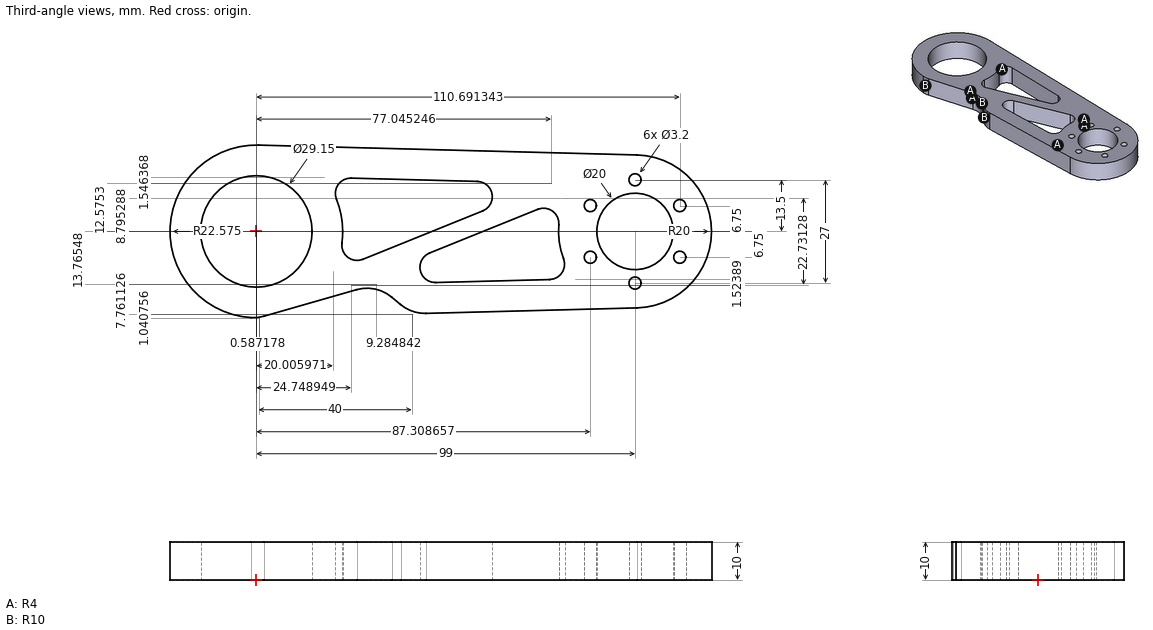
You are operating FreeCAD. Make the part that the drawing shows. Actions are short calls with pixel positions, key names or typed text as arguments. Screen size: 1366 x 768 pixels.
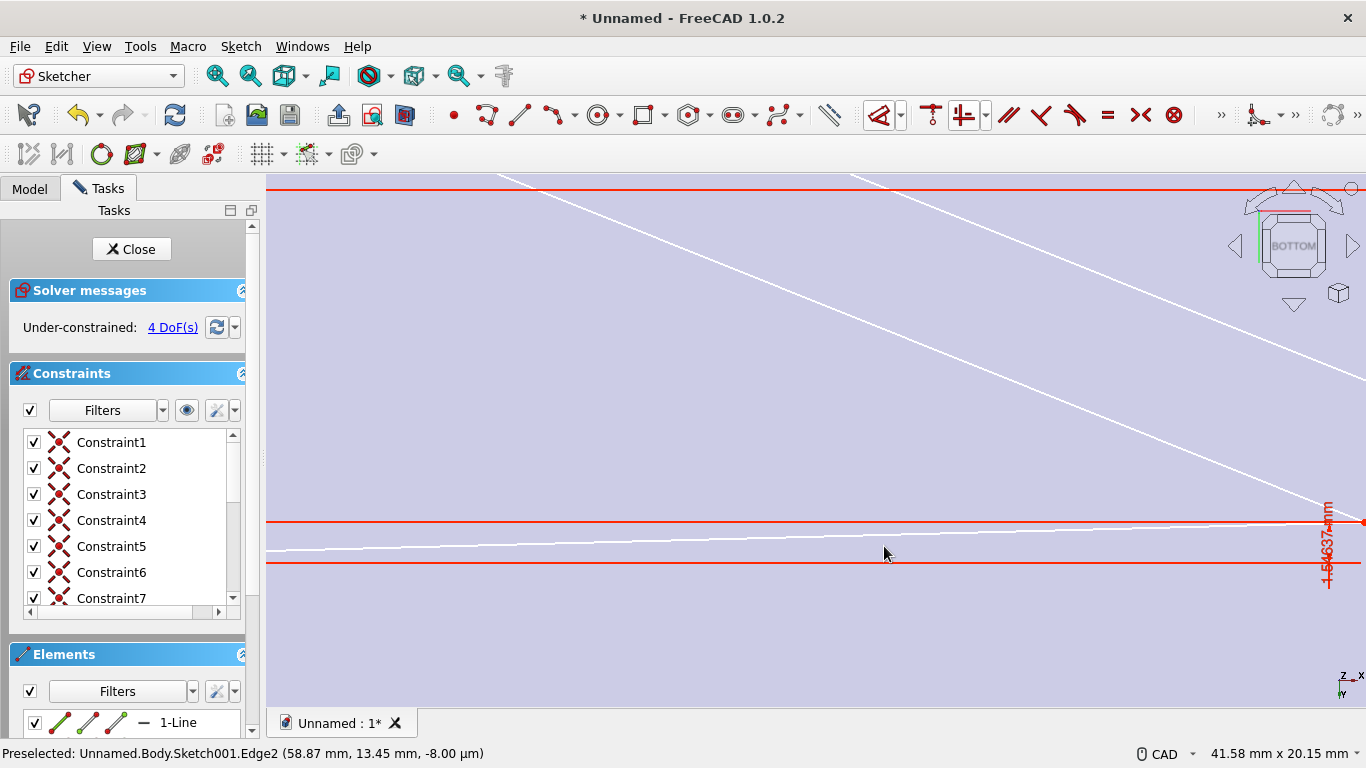
click(1023, 243)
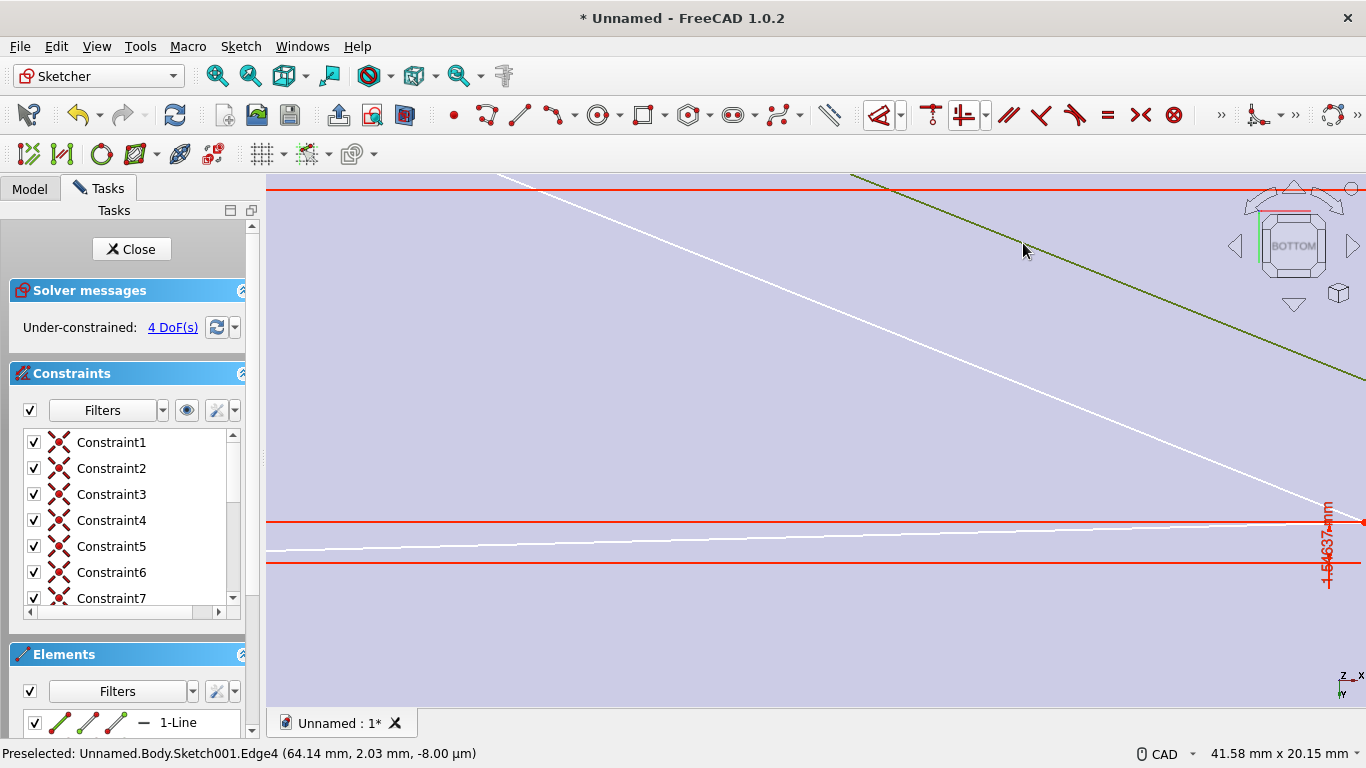
key(i)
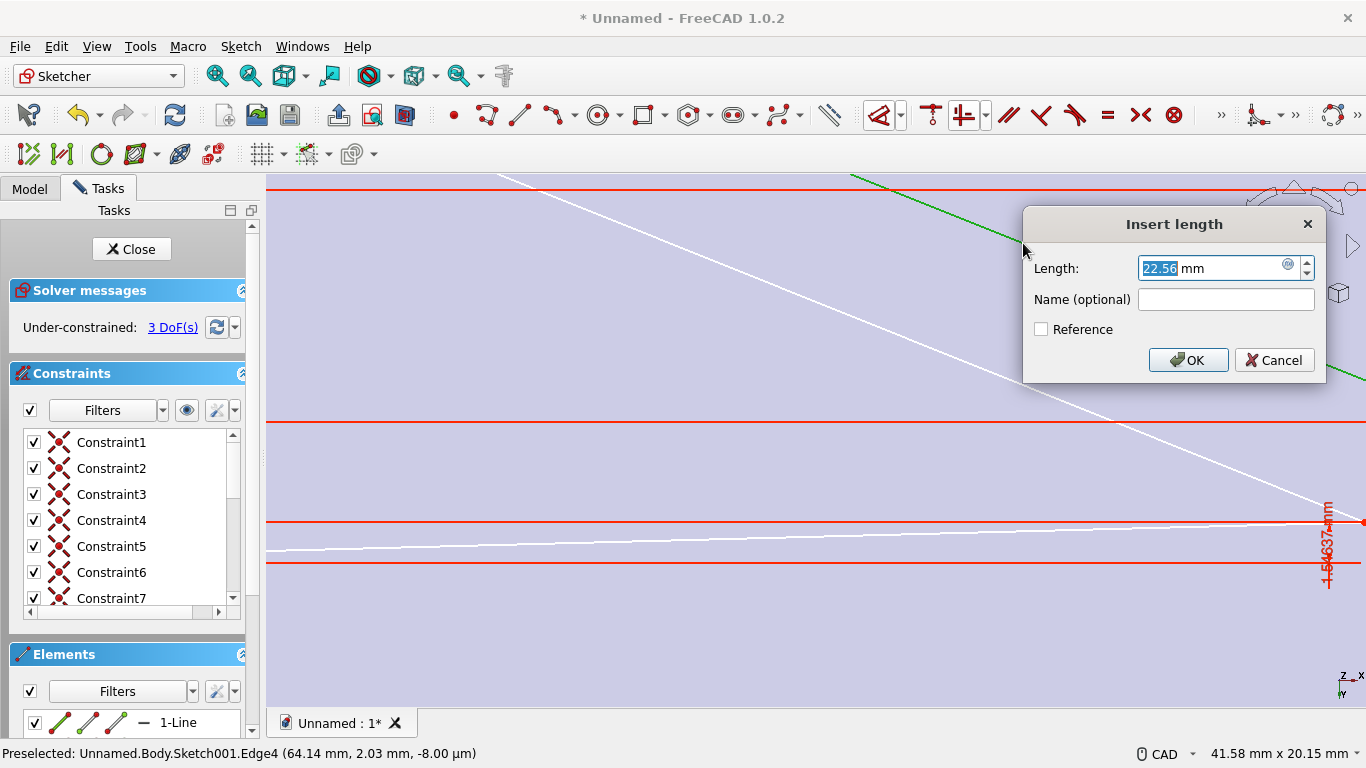
text(22.73128)
key(Return)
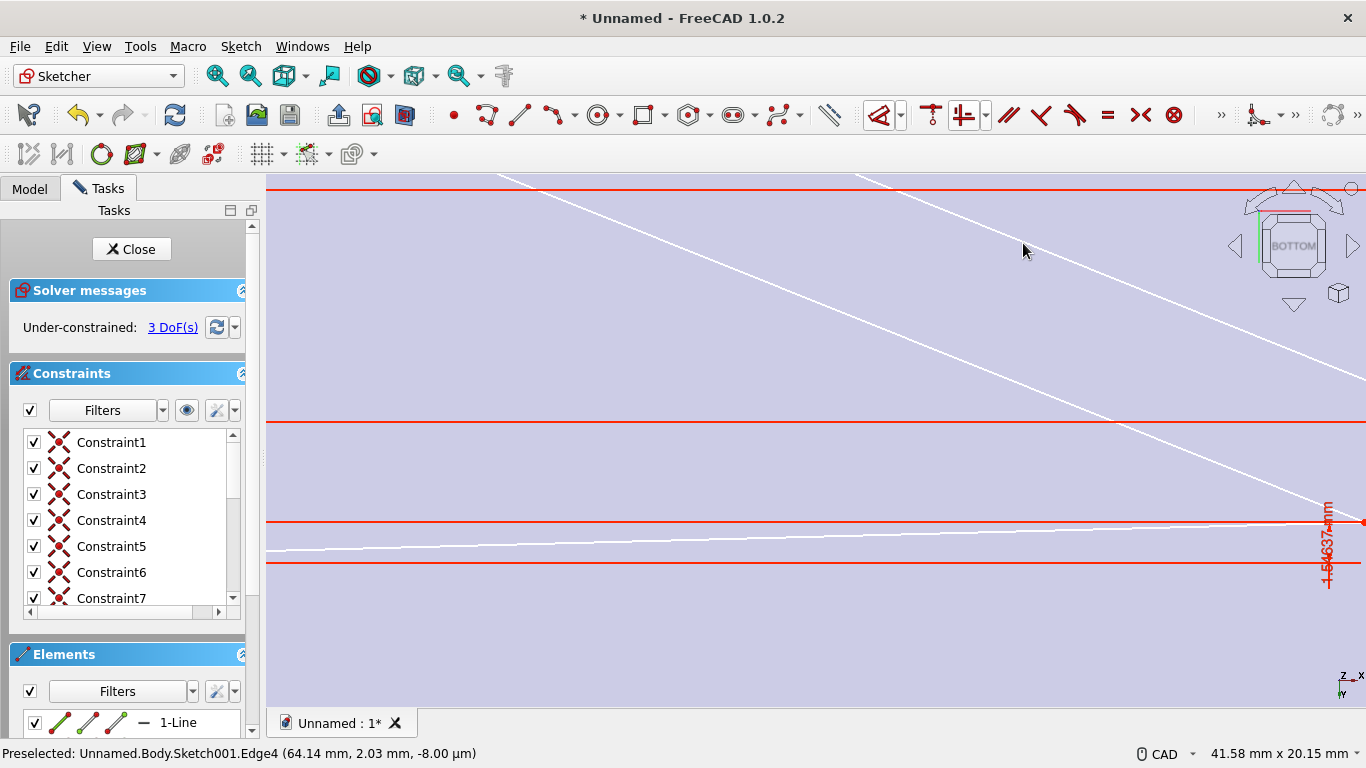
scroll(885, 548, down, 6)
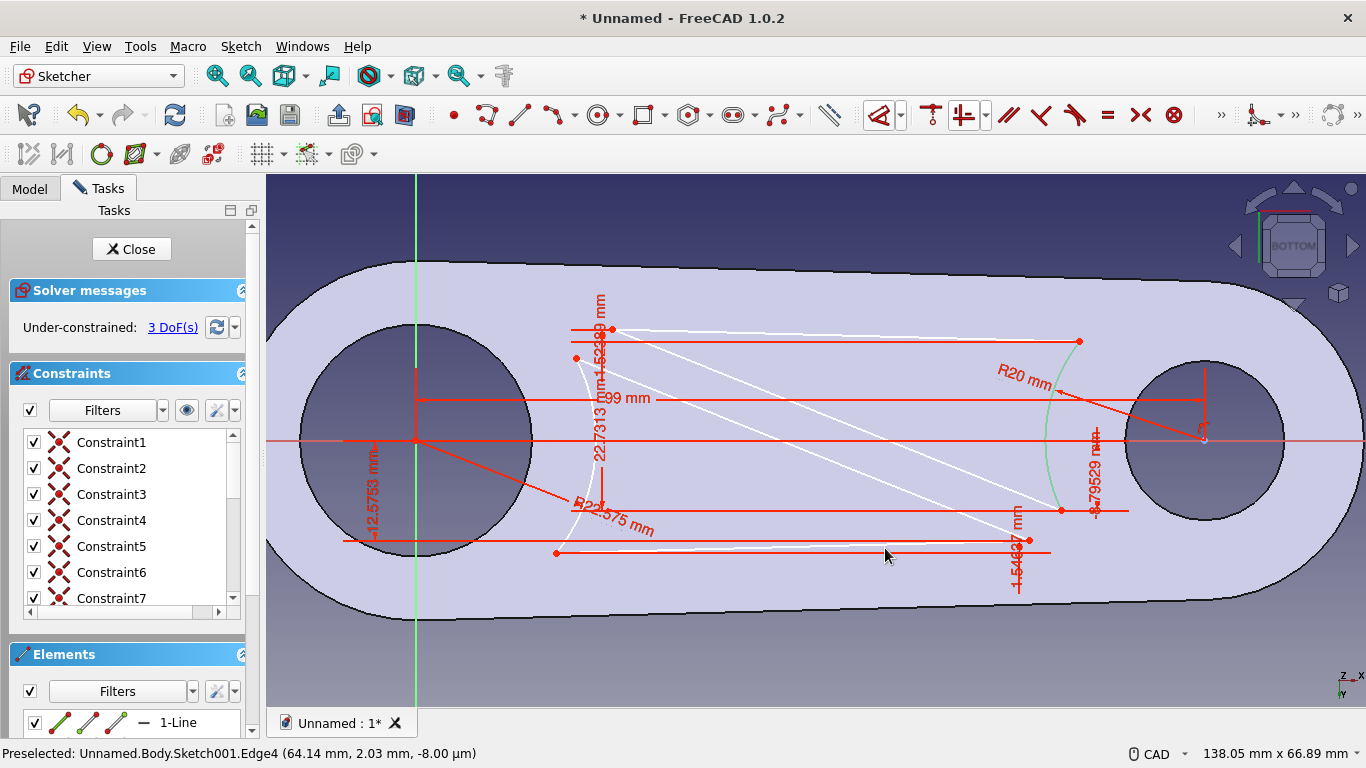
click(576, 358)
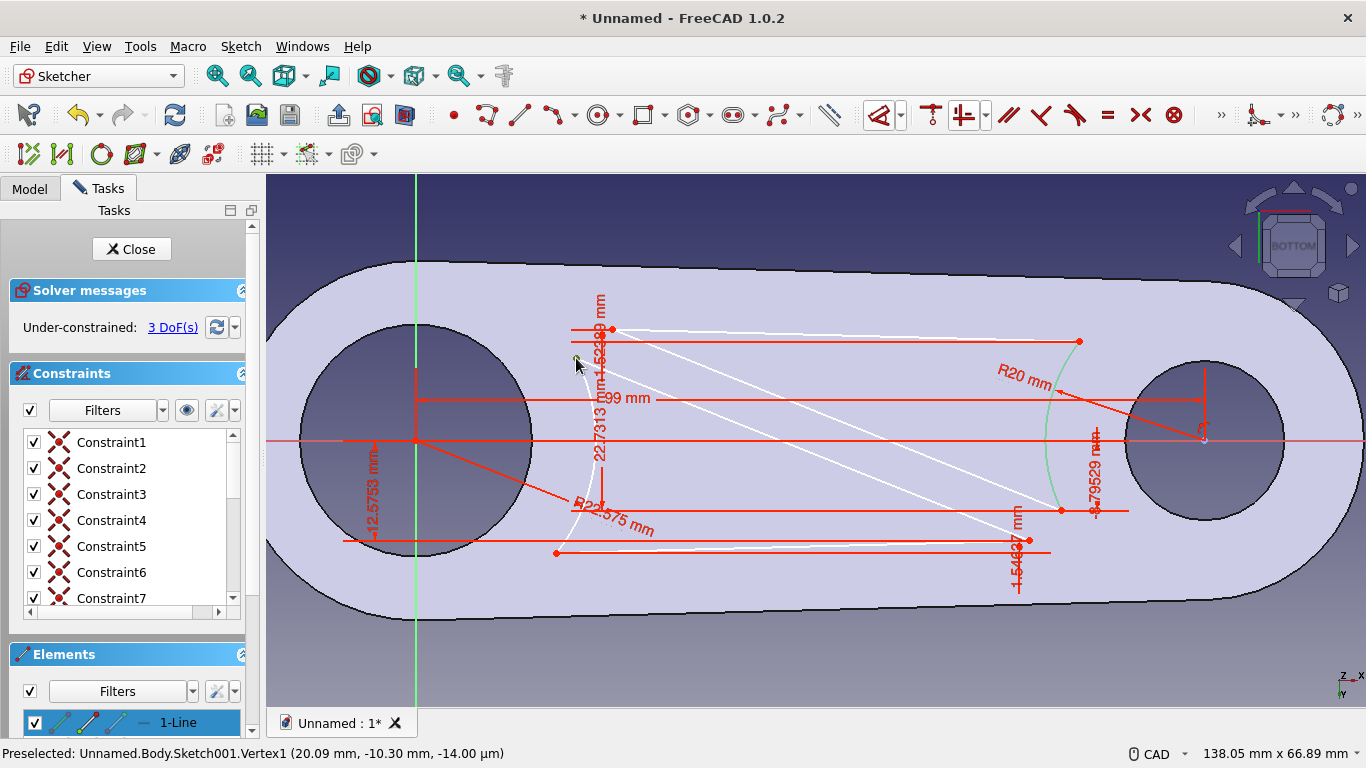
click(900, 116)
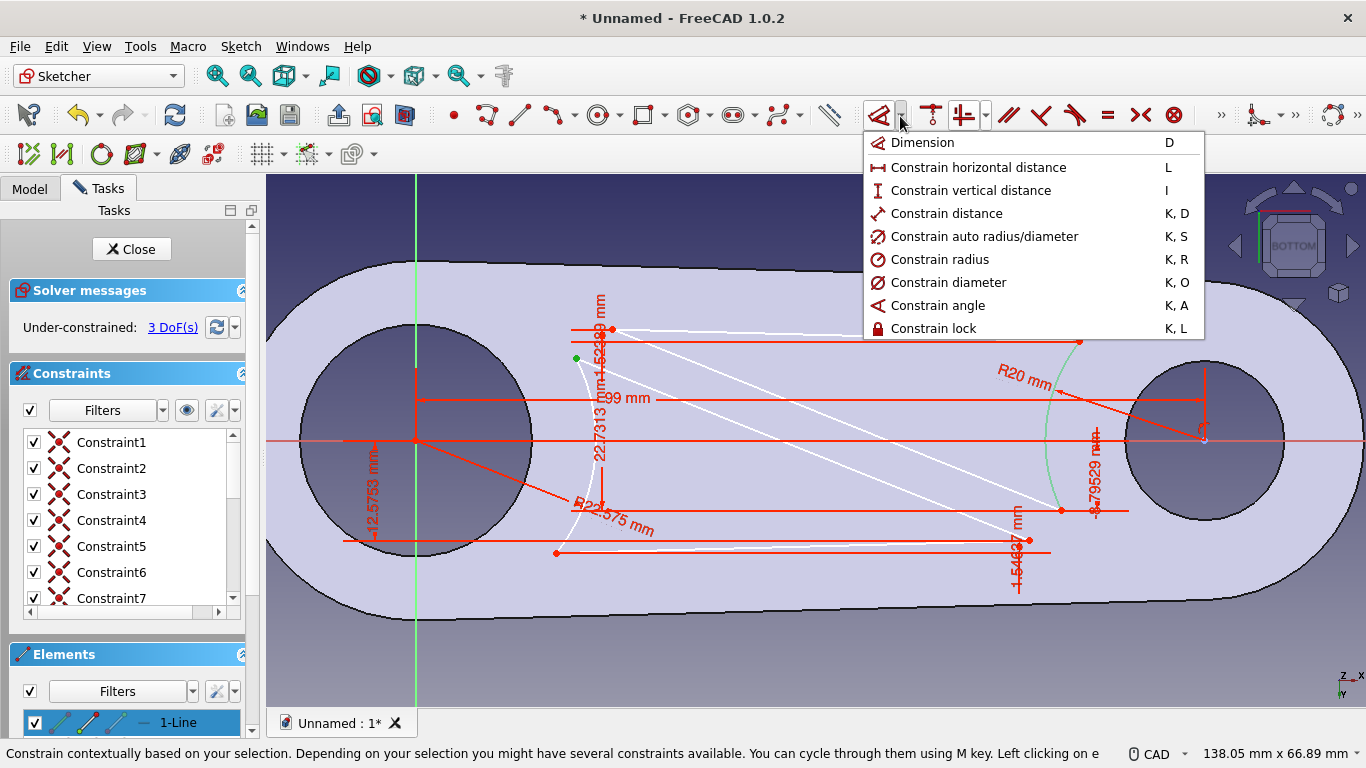
click(1034, 168)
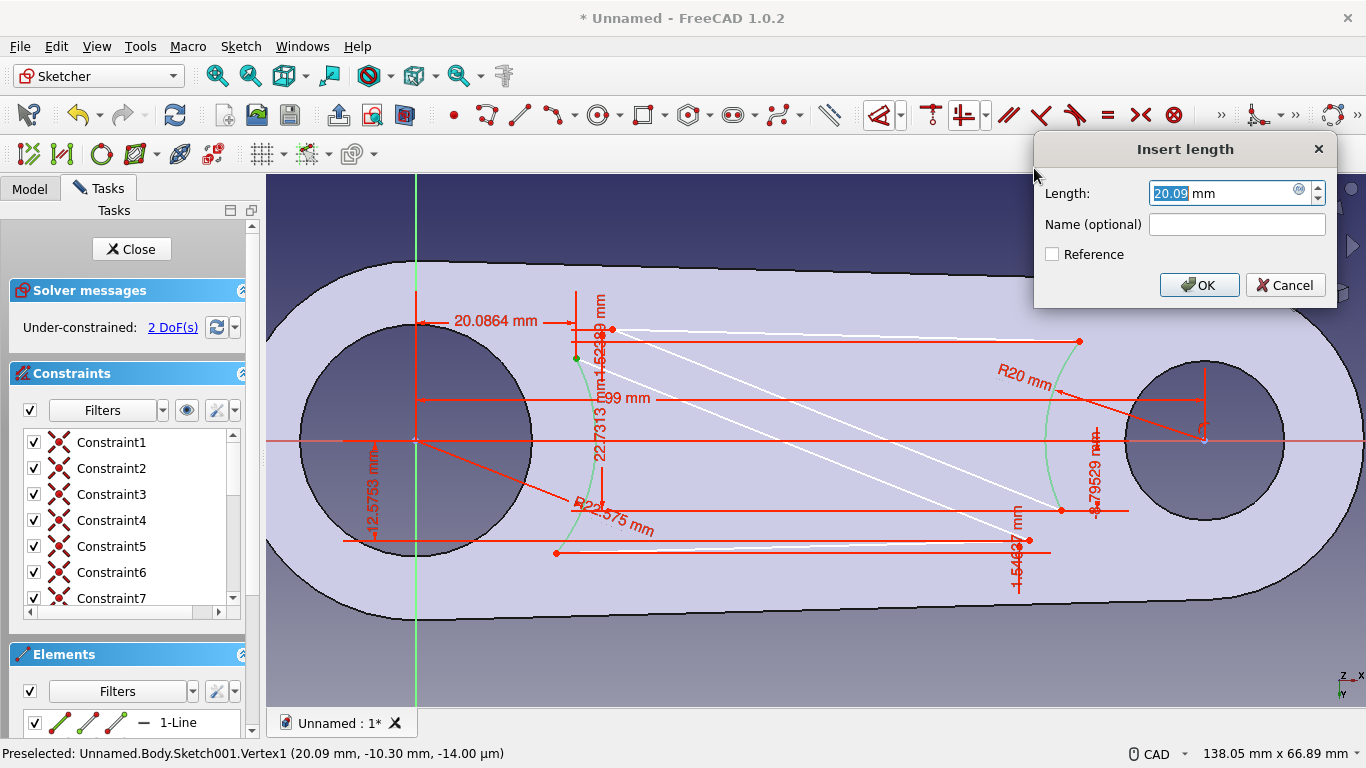
text(20.005971)
key(Return)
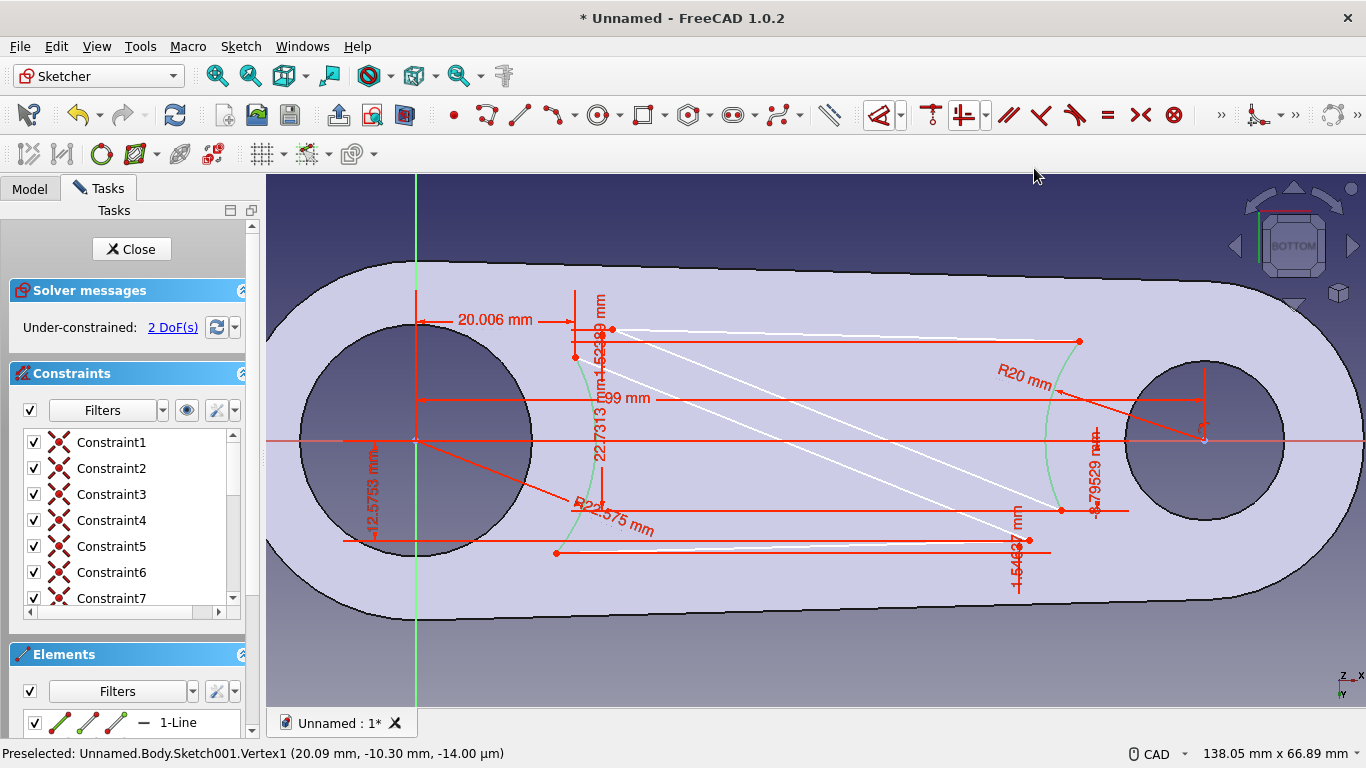
click(1030, 541)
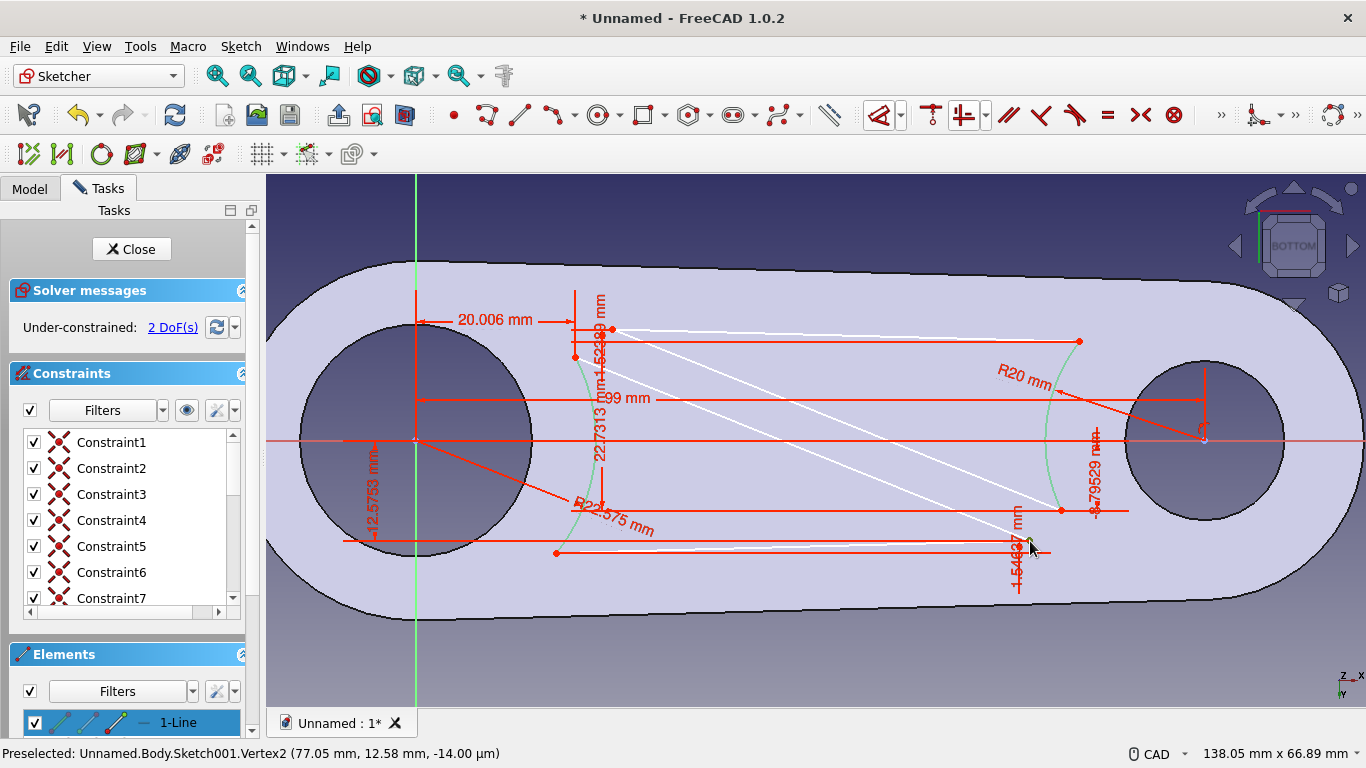
key(l)